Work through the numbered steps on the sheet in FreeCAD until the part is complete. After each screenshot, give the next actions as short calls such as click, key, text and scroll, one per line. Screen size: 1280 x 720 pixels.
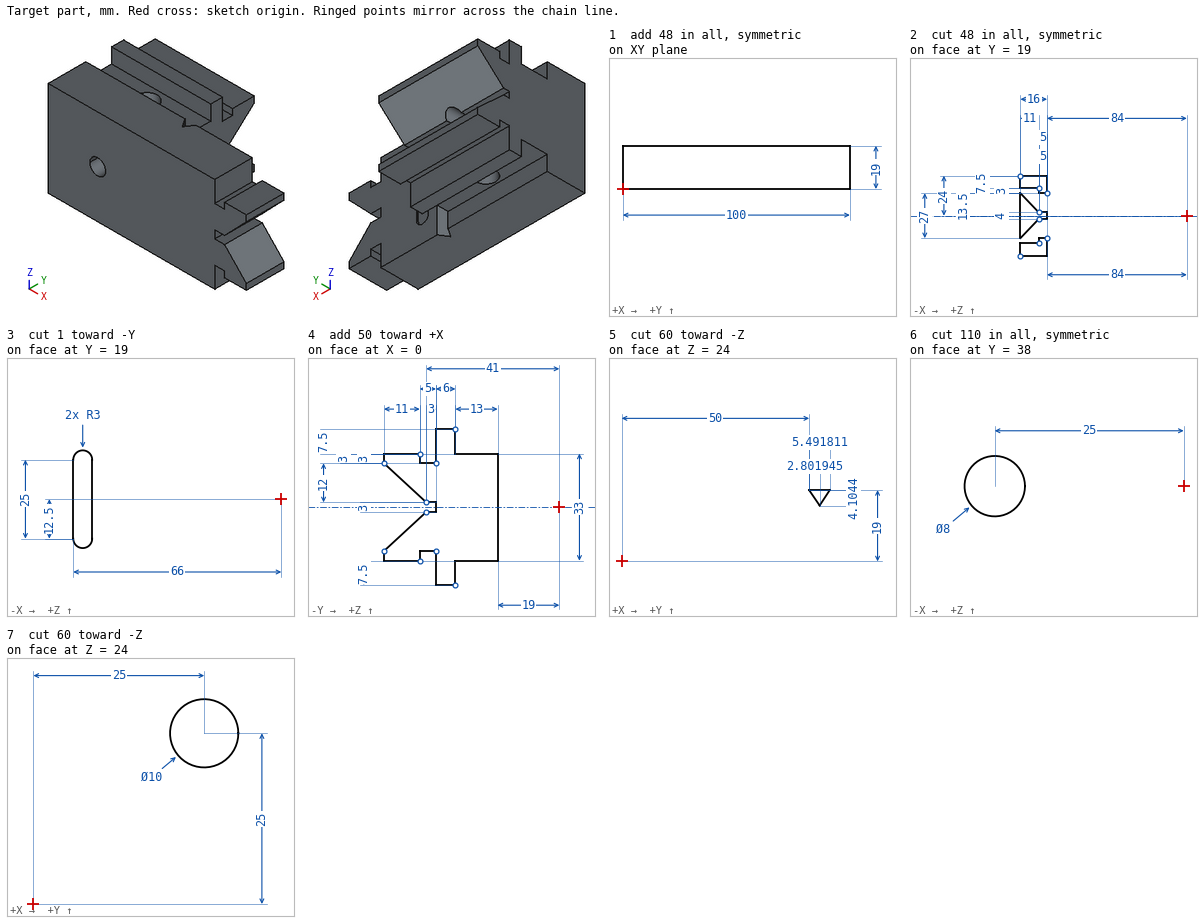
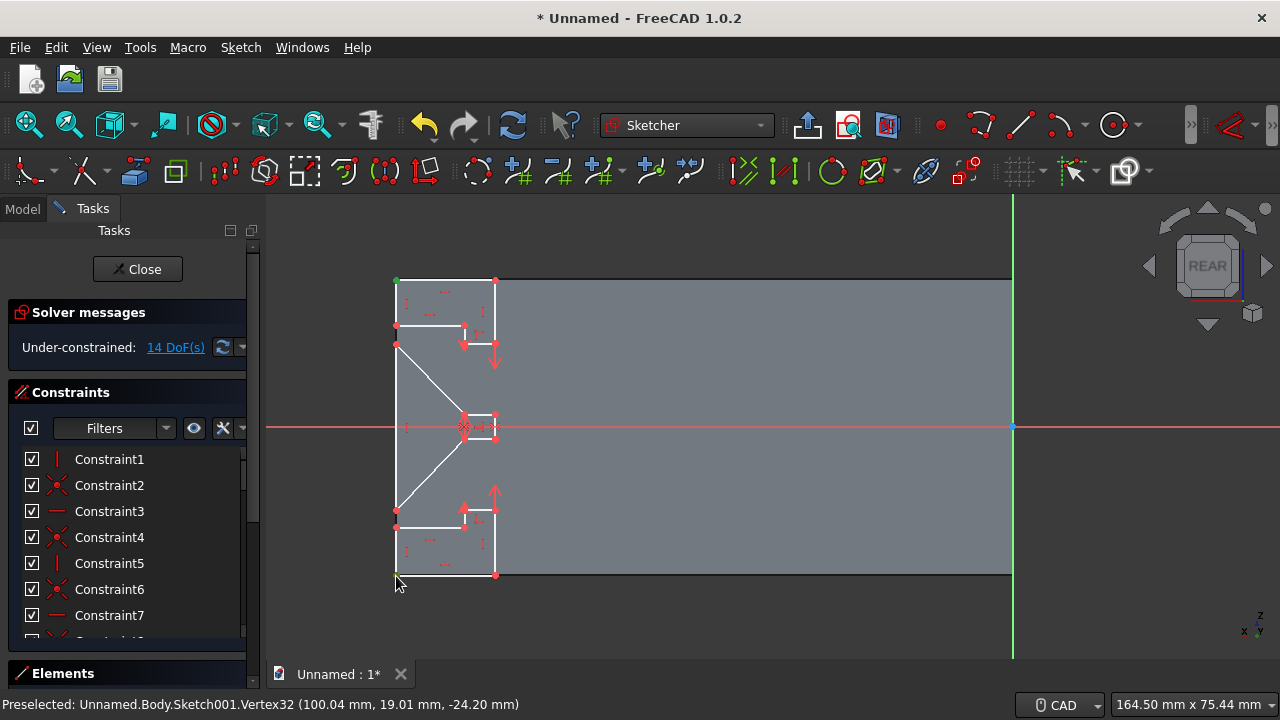
click(353, 427)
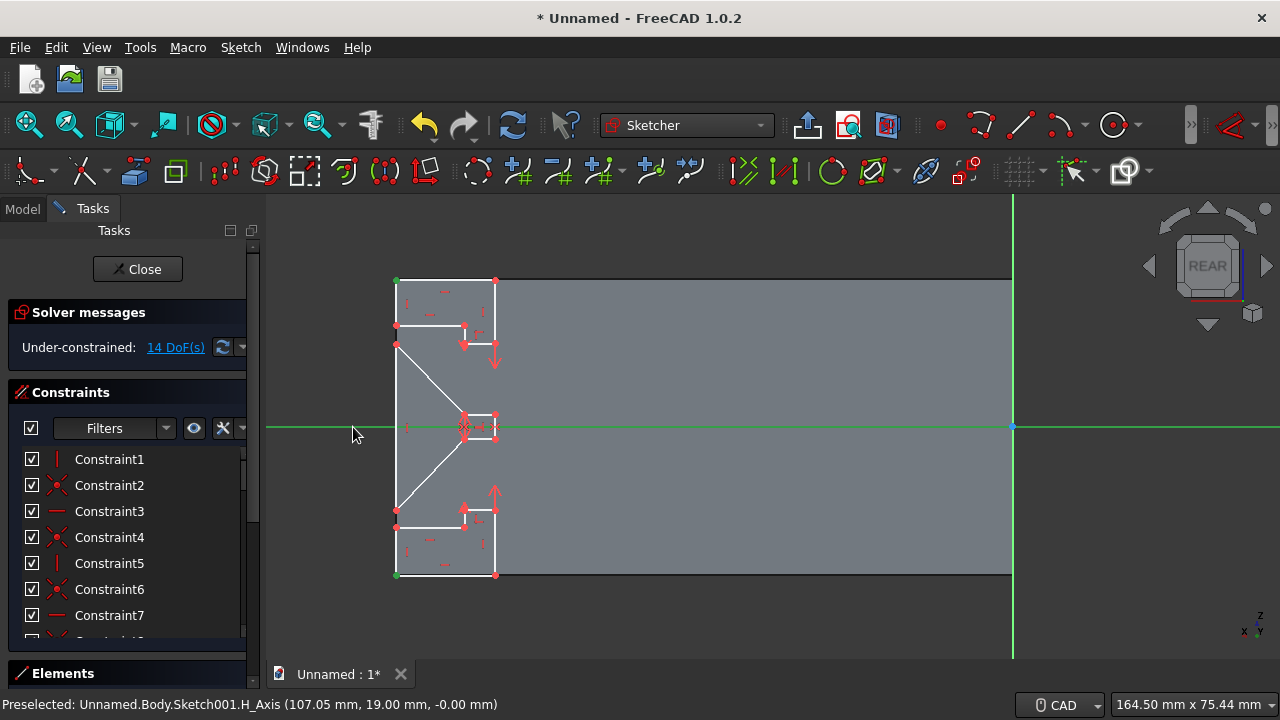
key(s)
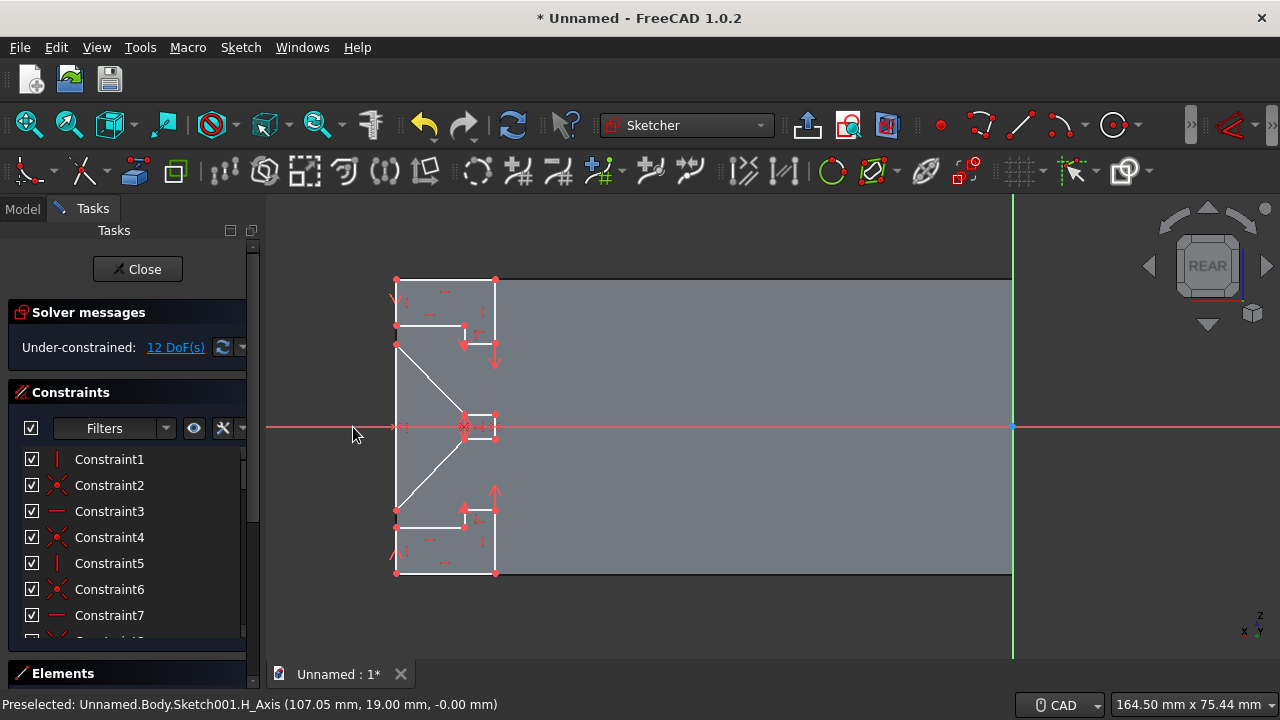
click(1230, 126)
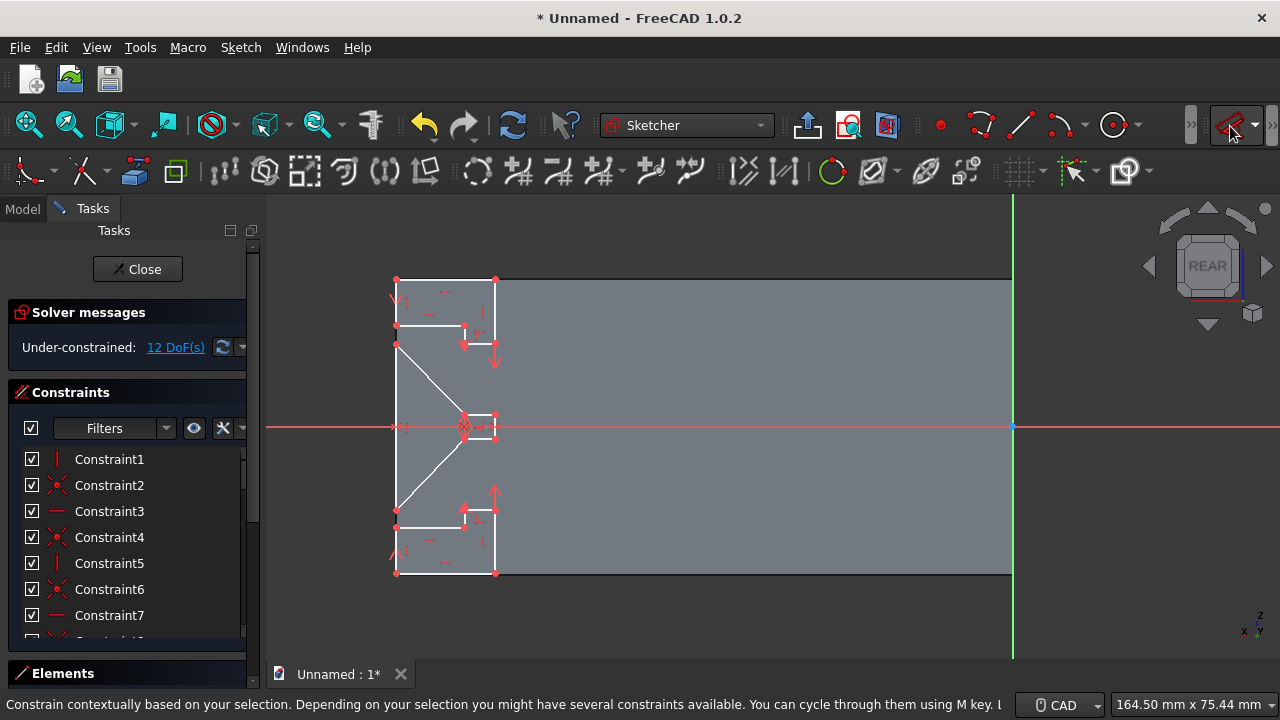
scroll(465, 335, up, 4)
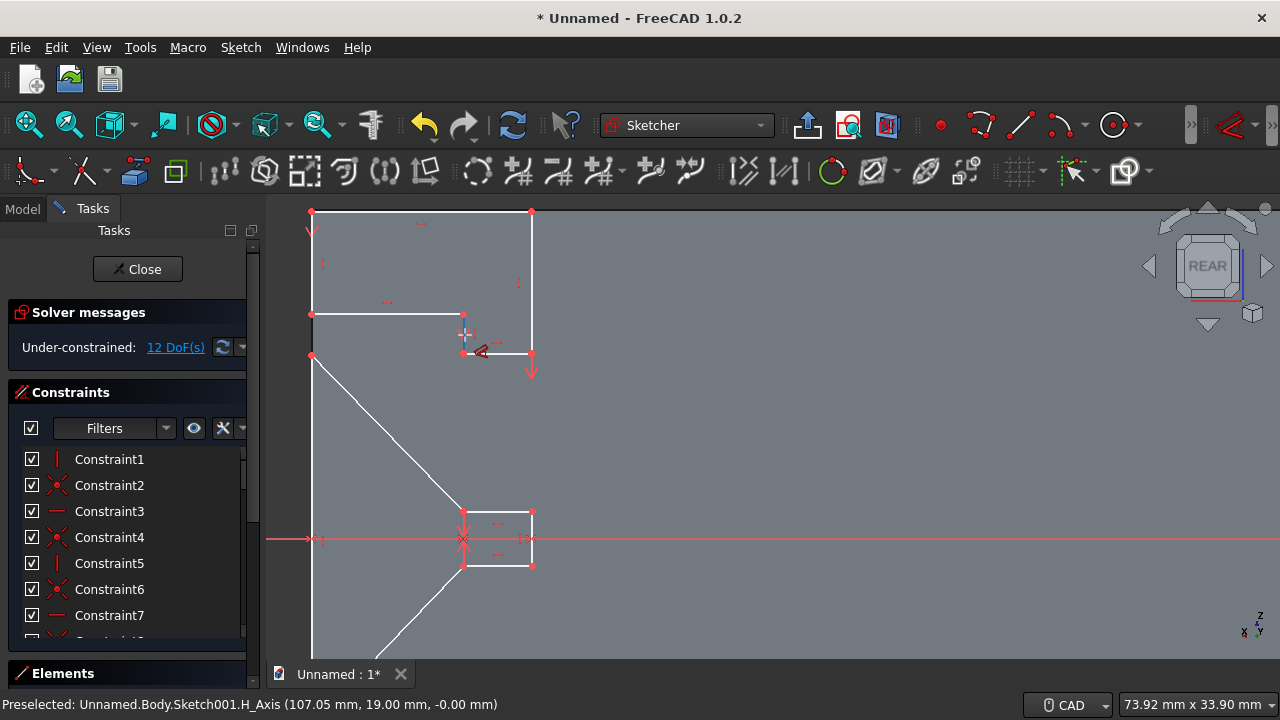
click(464, 334)
click(430, 334)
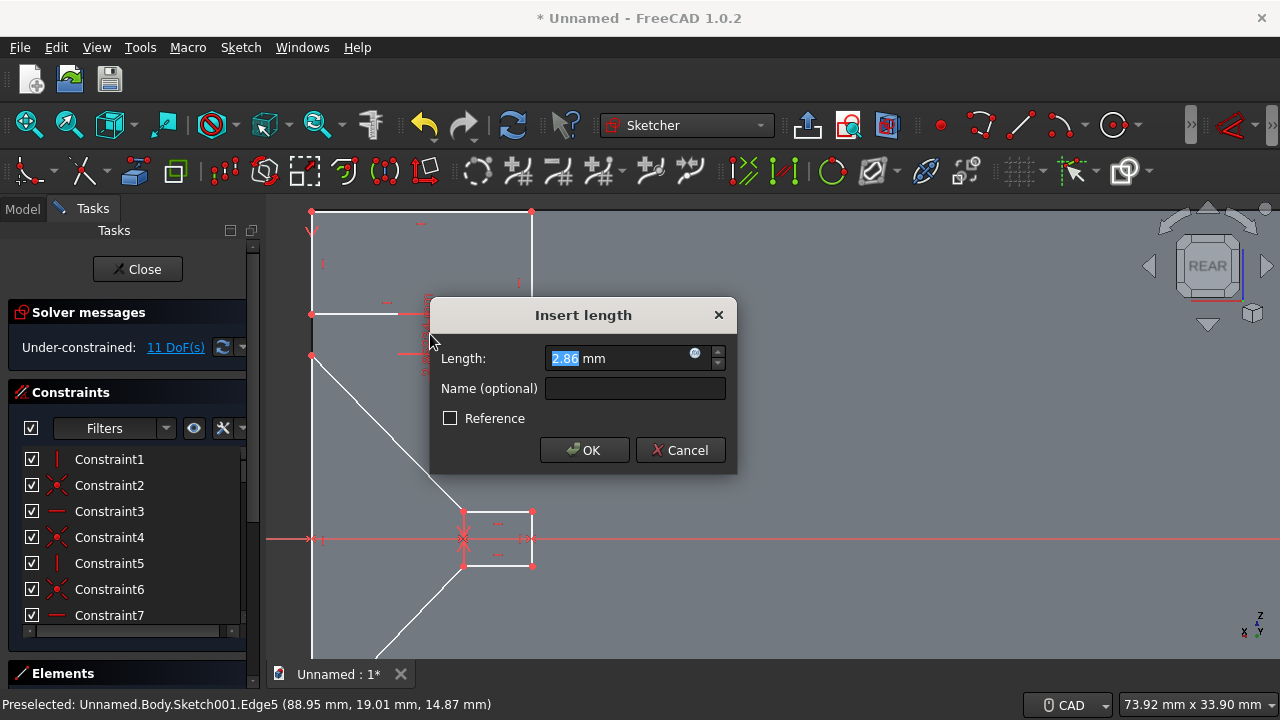
text(3)
key(Return)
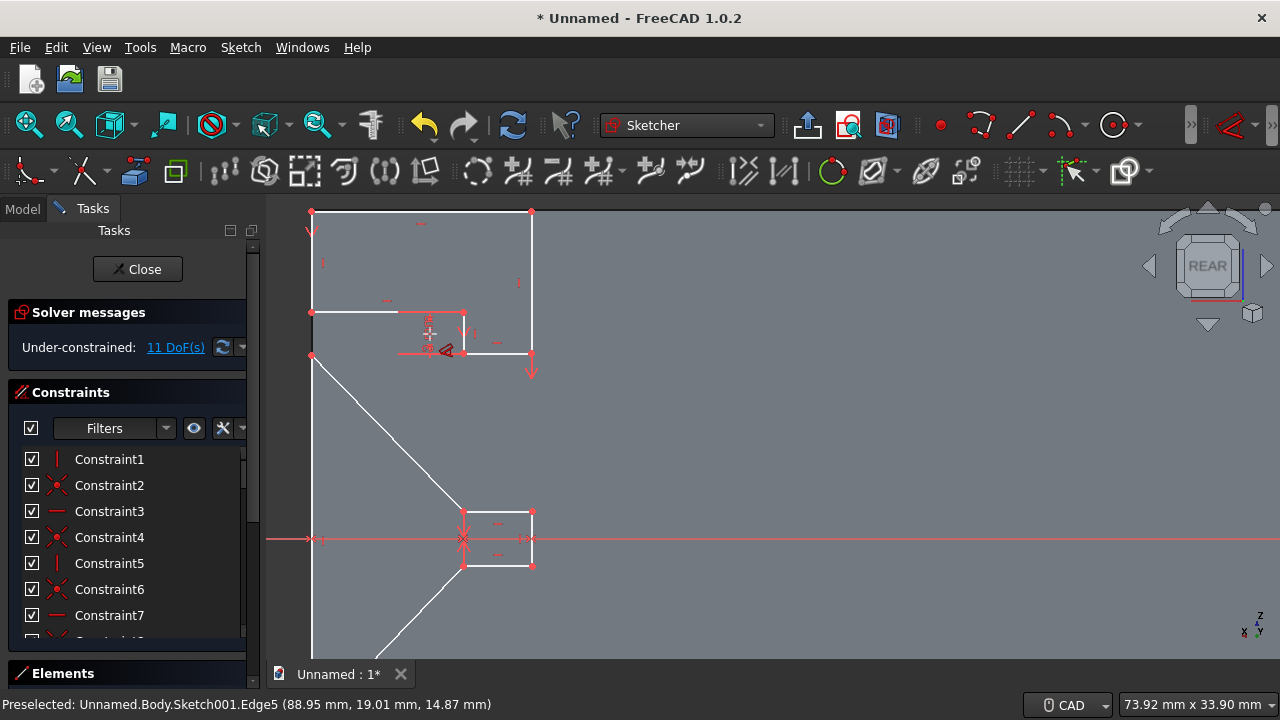
click(484, 354)
click(513, 320)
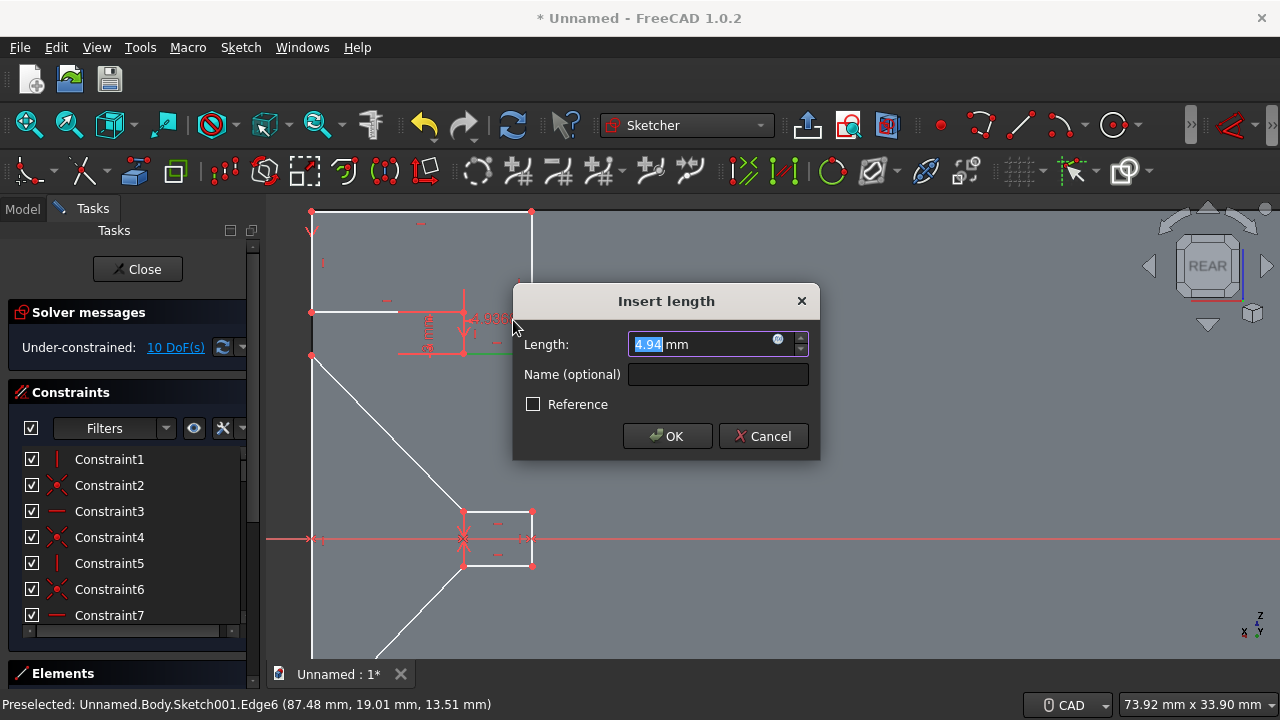
text(5)
key(Return)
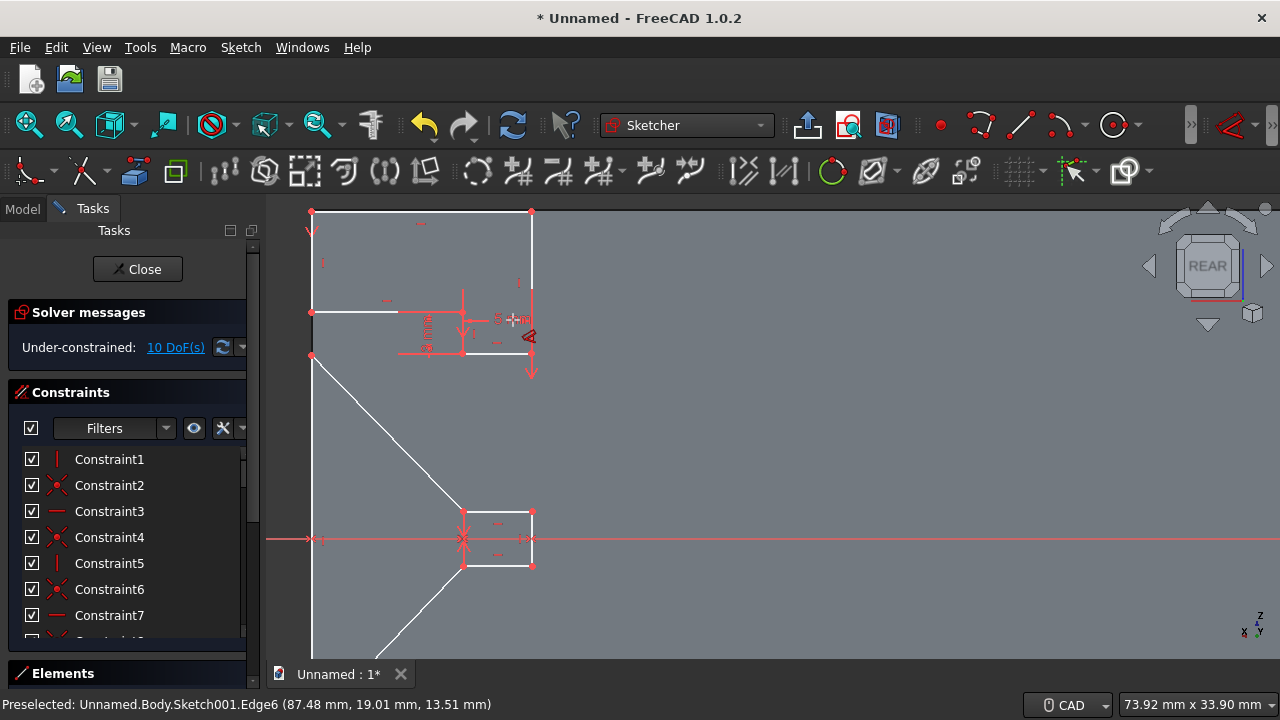
scroll(532, 550, up, 2)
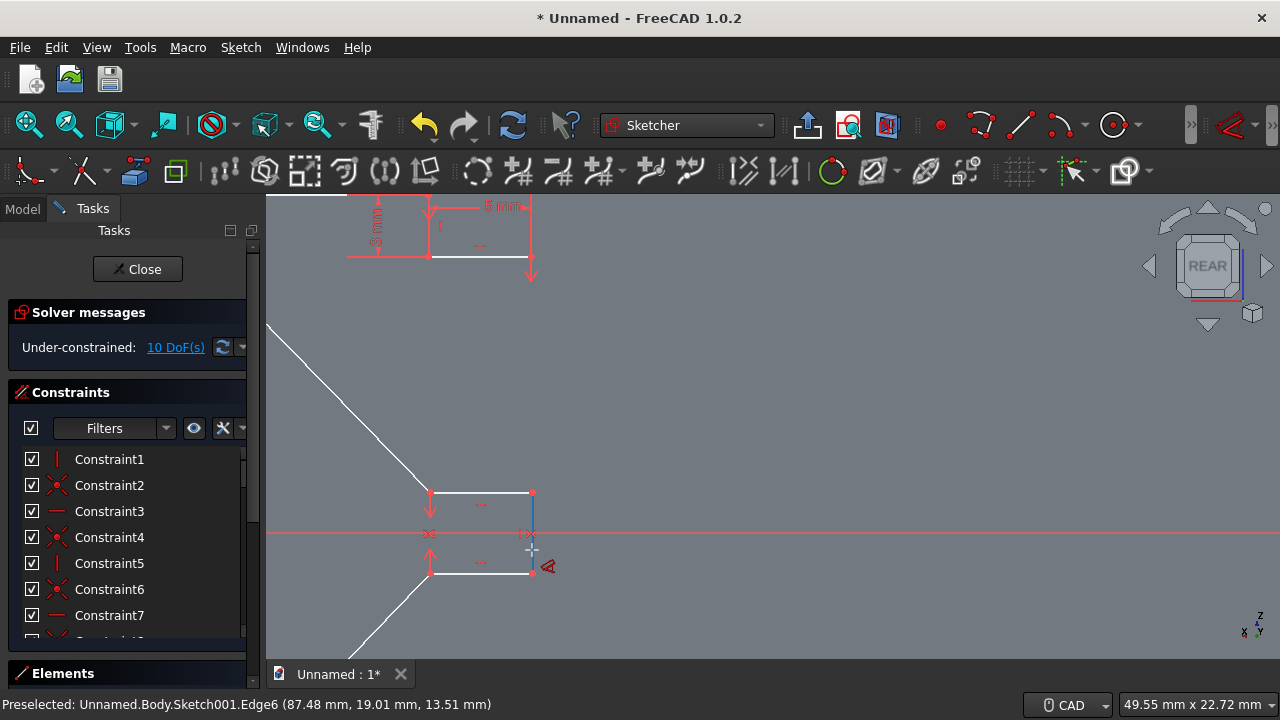
click(533, 549)
click(499, 515)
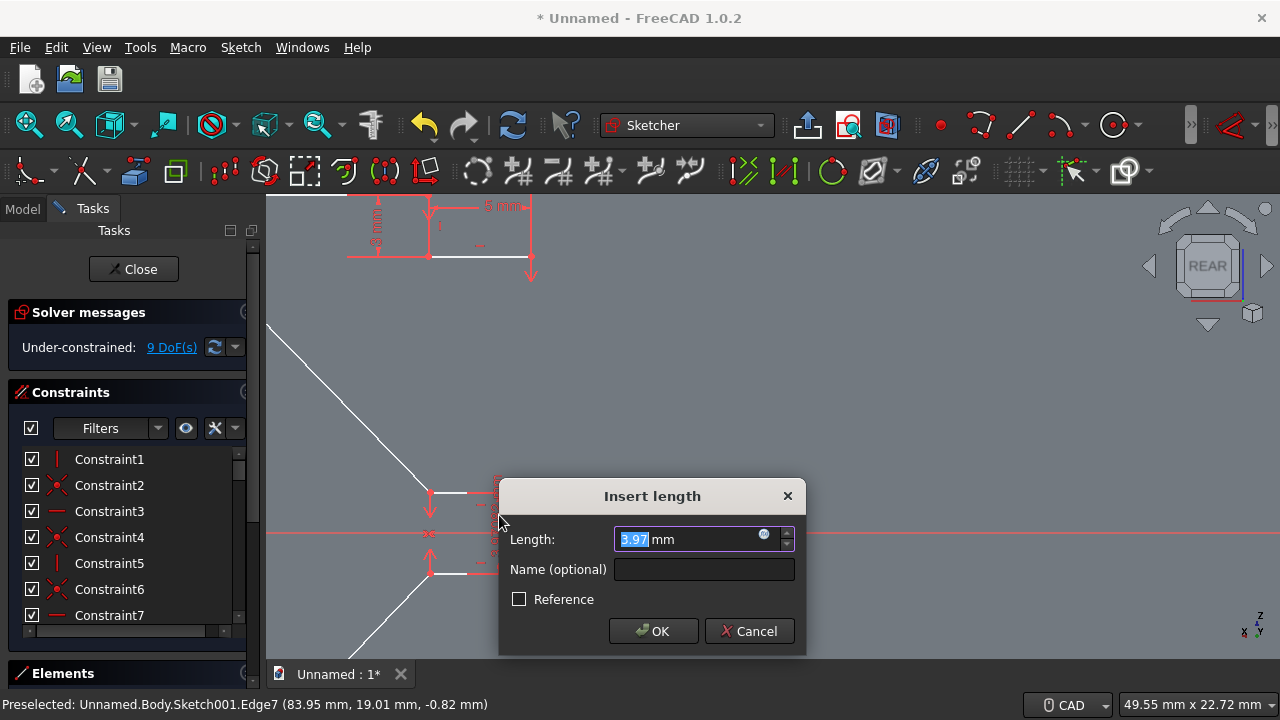
text(4)
key(Return)